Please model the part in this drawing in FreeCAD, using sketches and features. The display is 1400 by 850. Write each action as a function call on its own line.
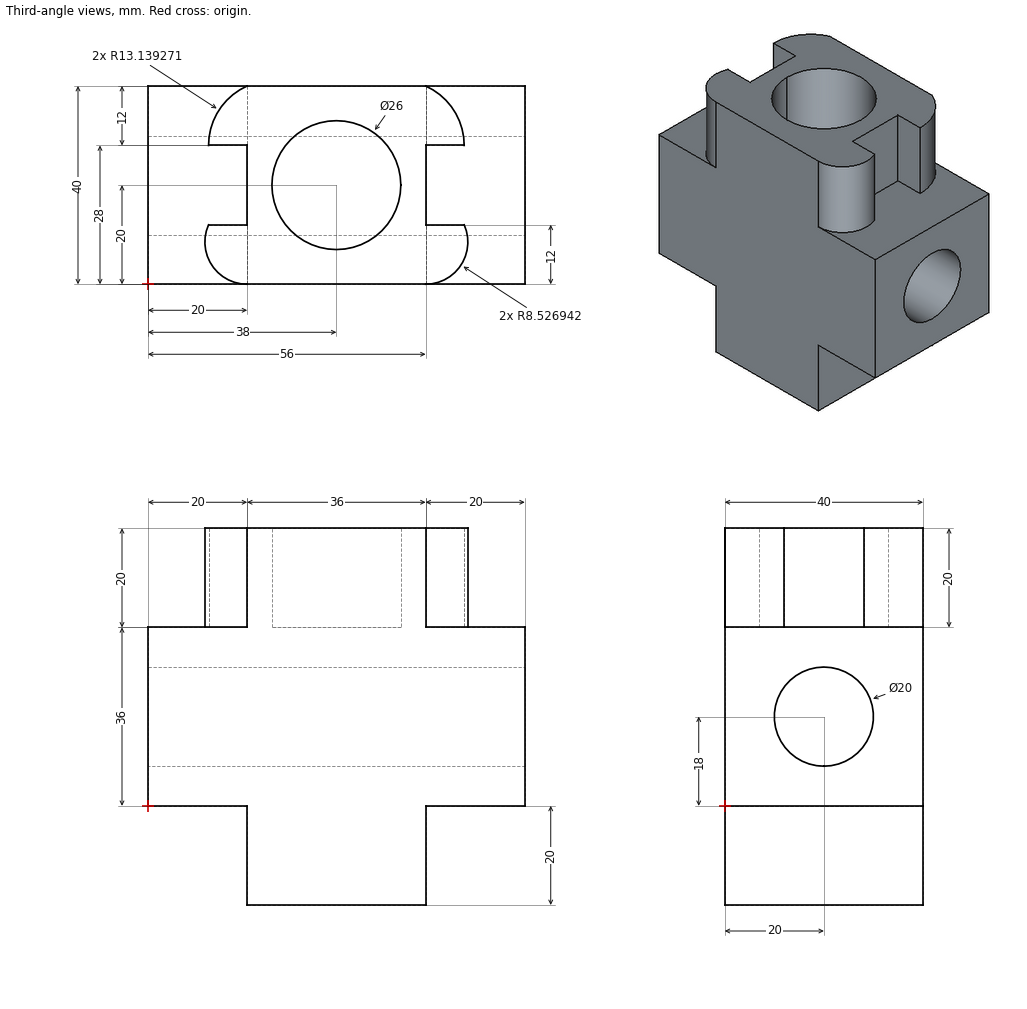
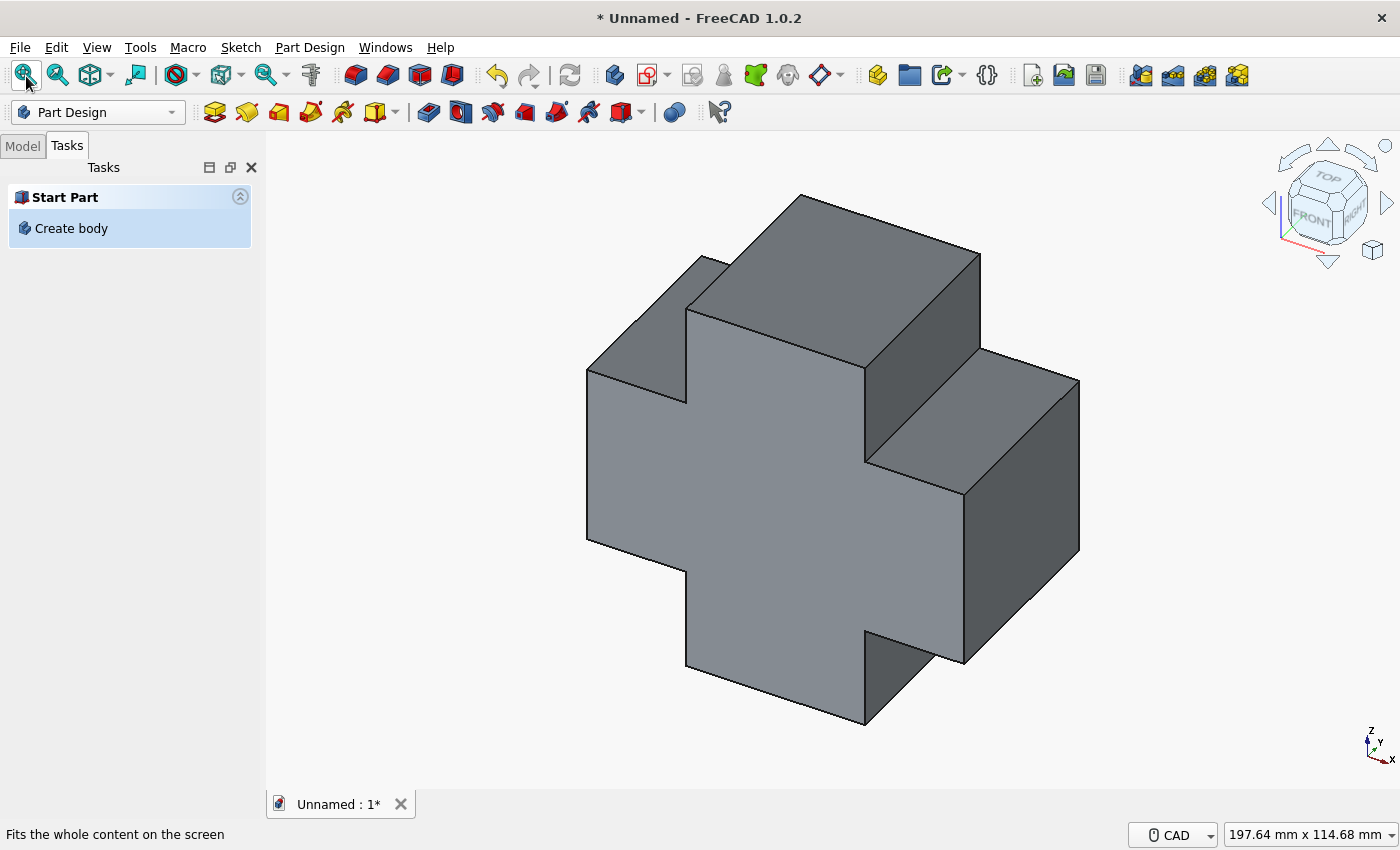
click(833, 280)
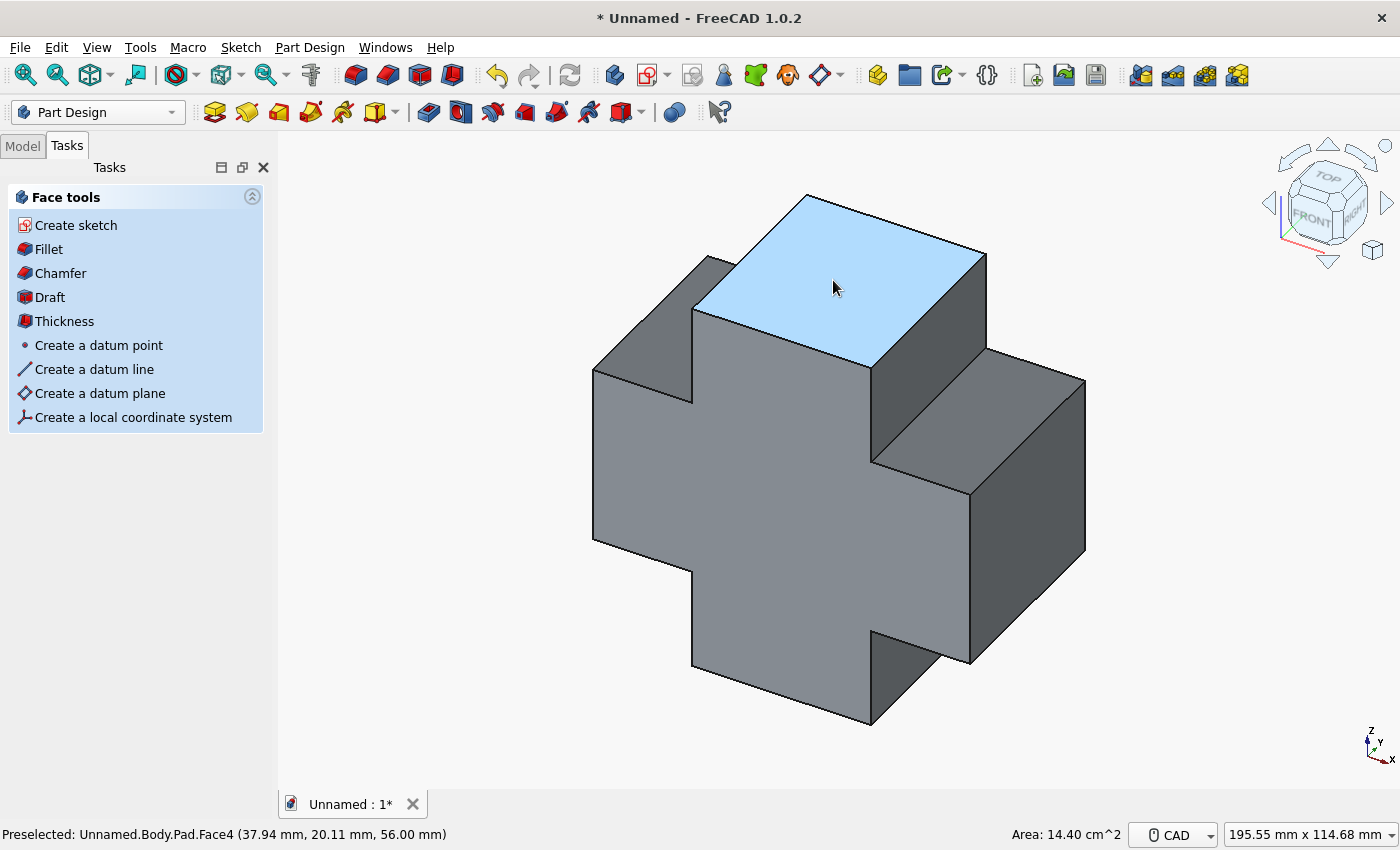
click(648, 76)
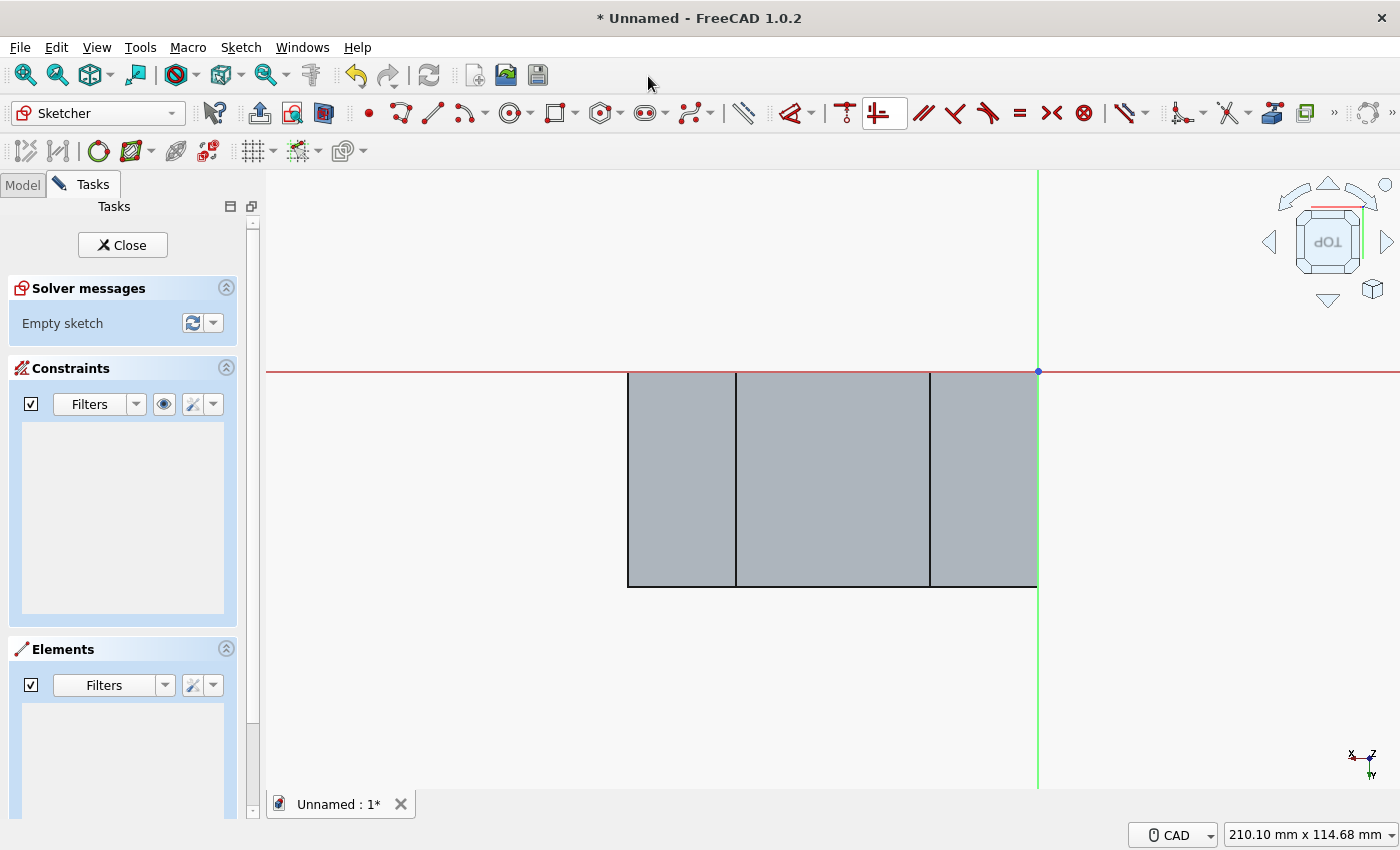
scroll(989, 480, up, 3)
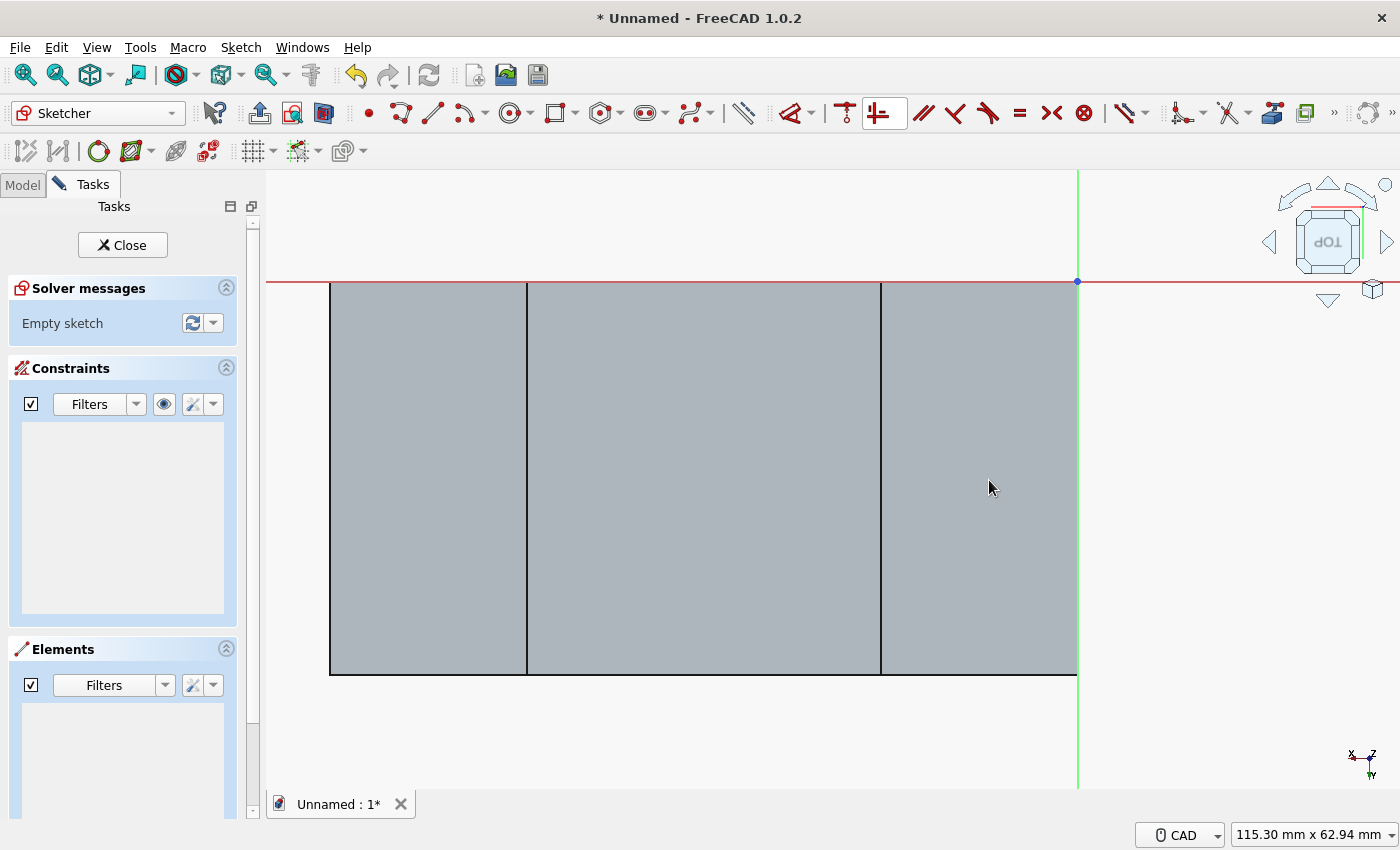
click(402, 114)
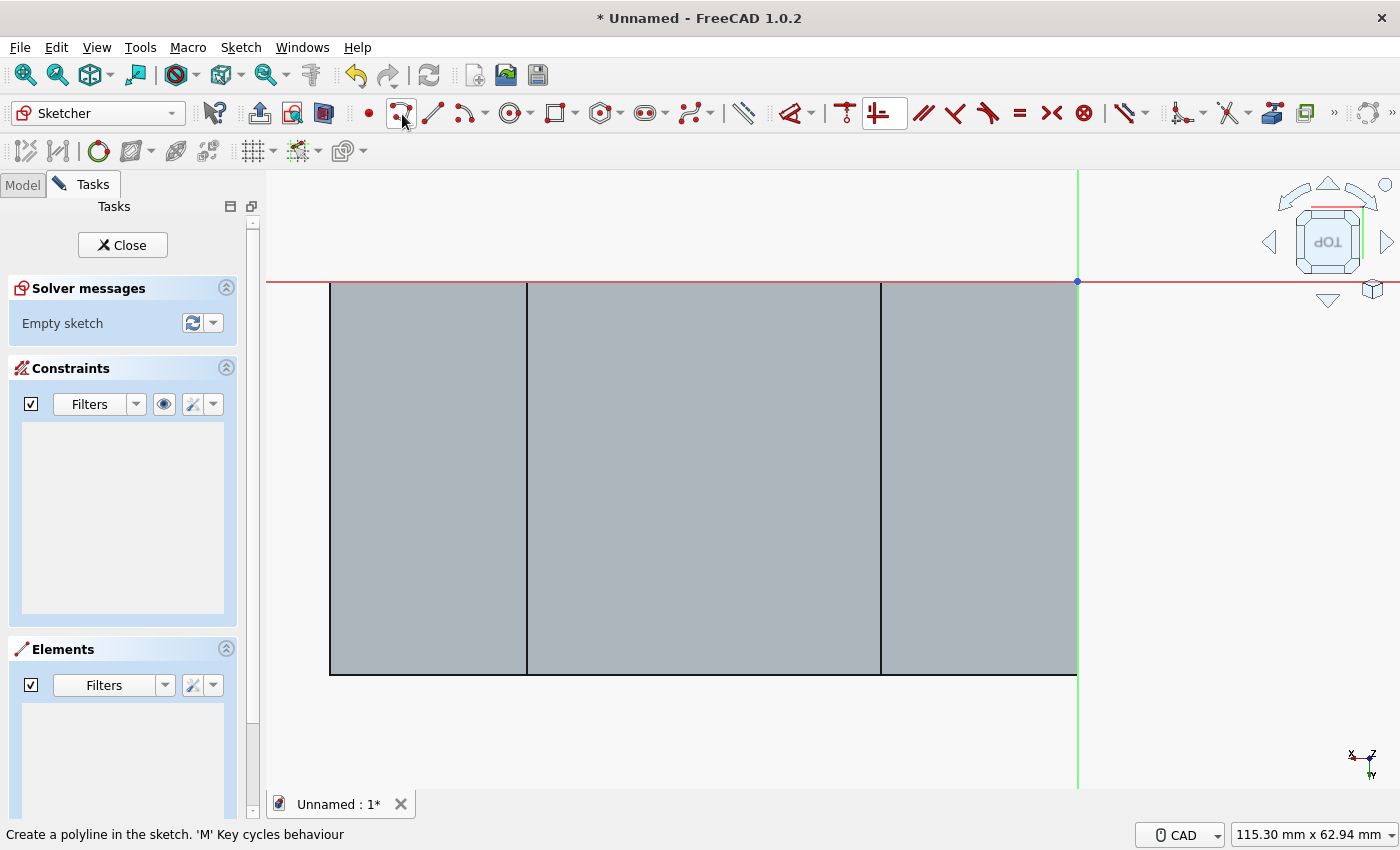
click(958, 557)
click(881, 557)
click(881, 675)
right_click(881, 675)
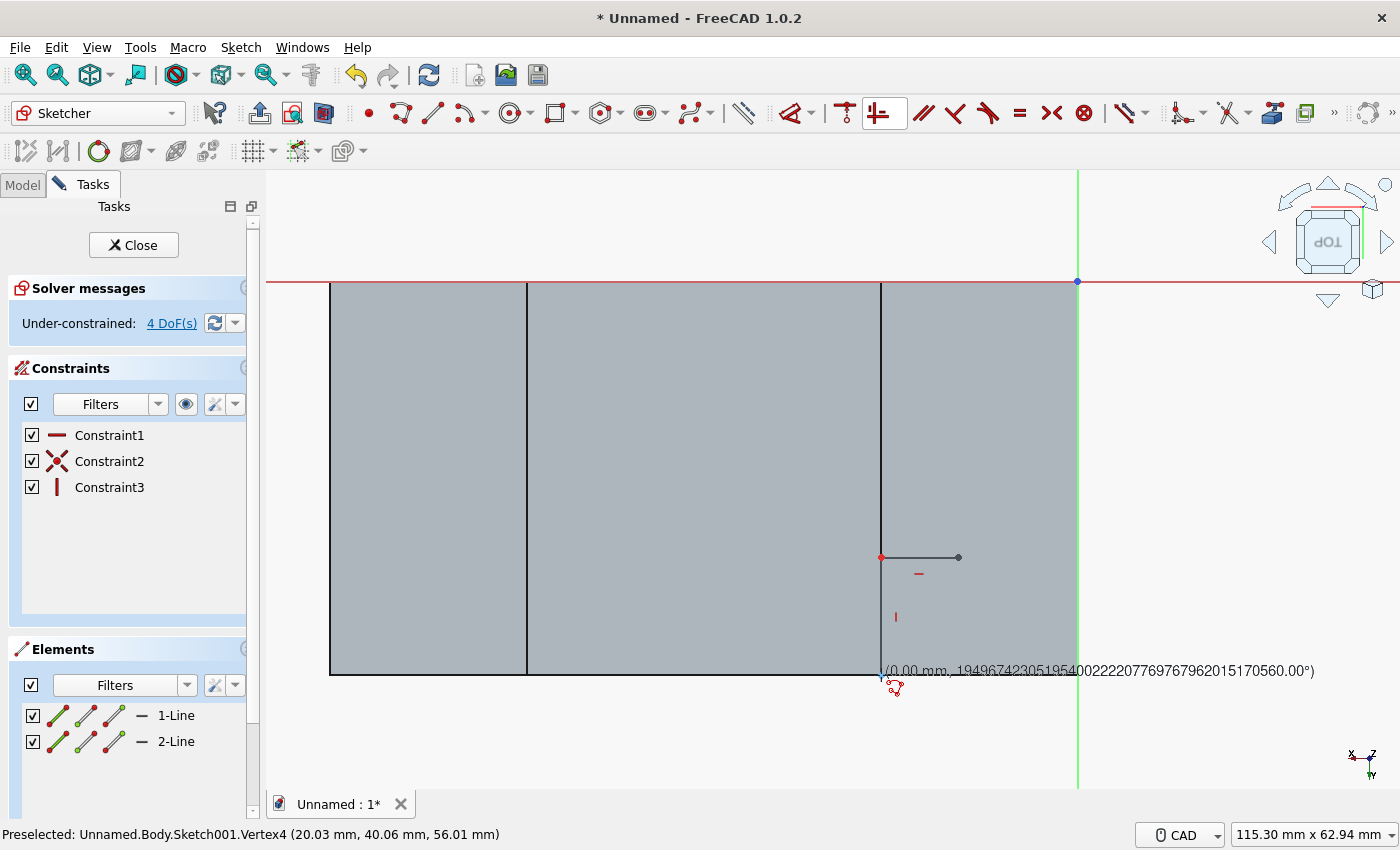
key(g)
key(3)
key(a)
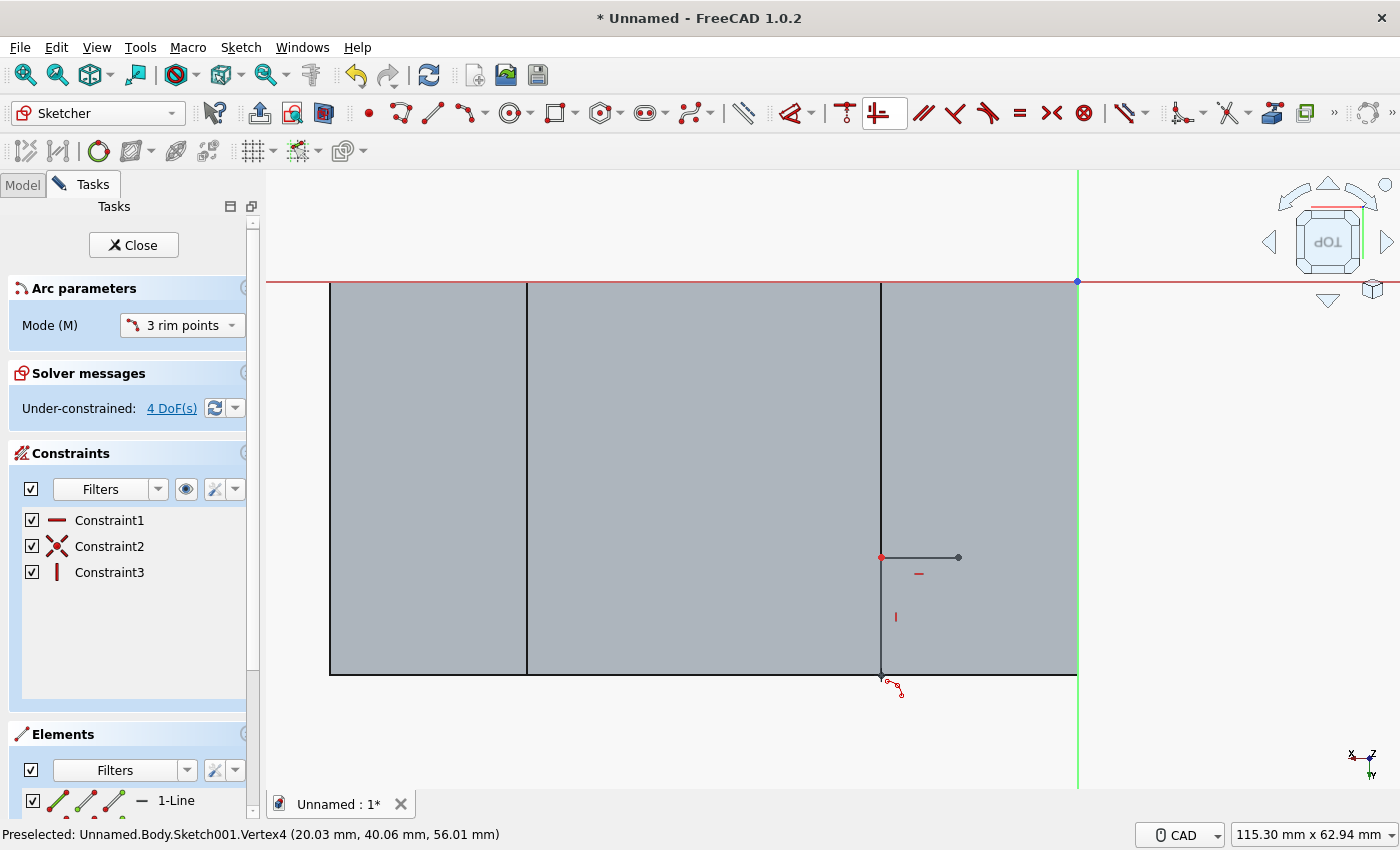
click(881, 676)
click(958, 558)
click(937, 628)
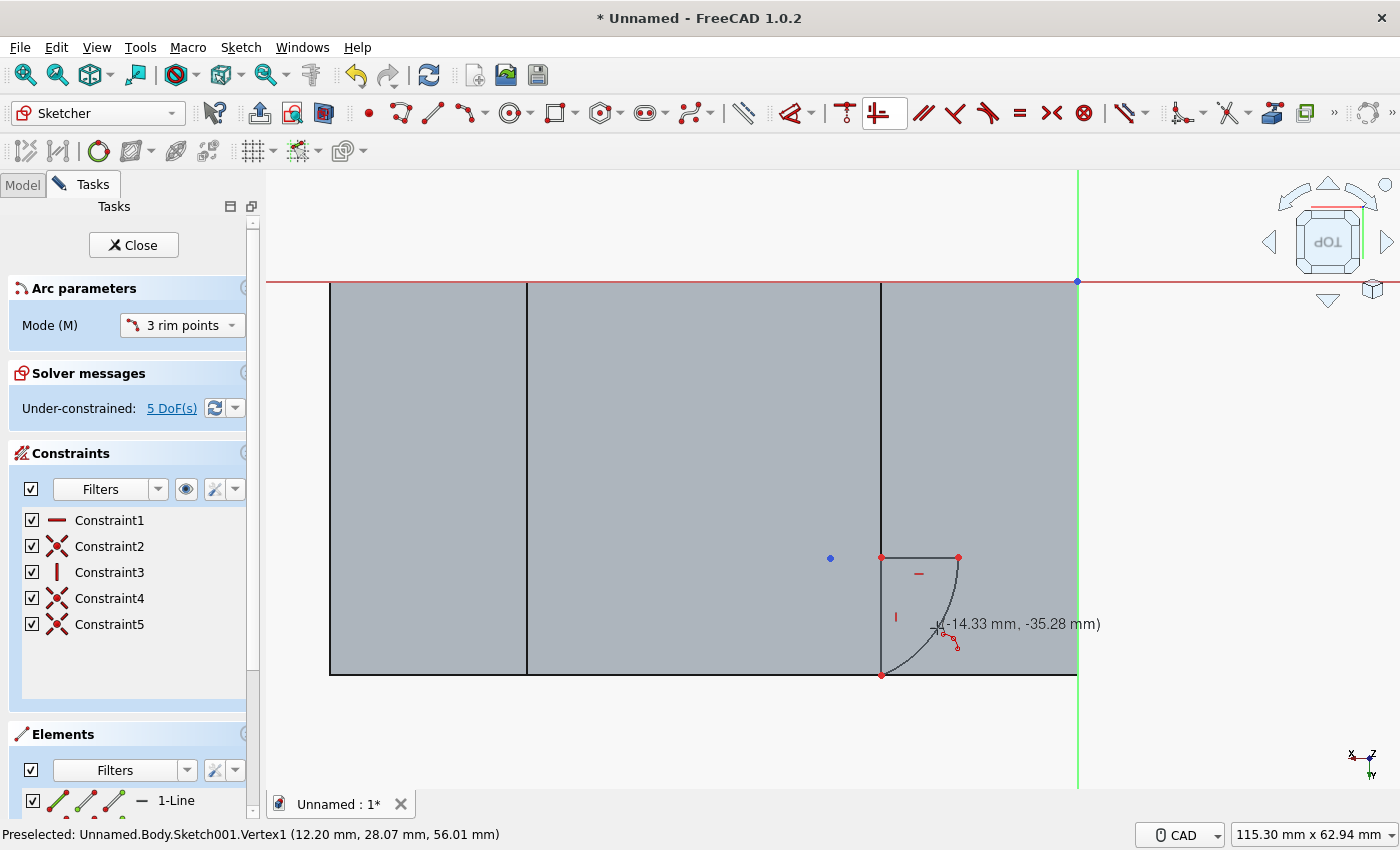
click(402, 114)